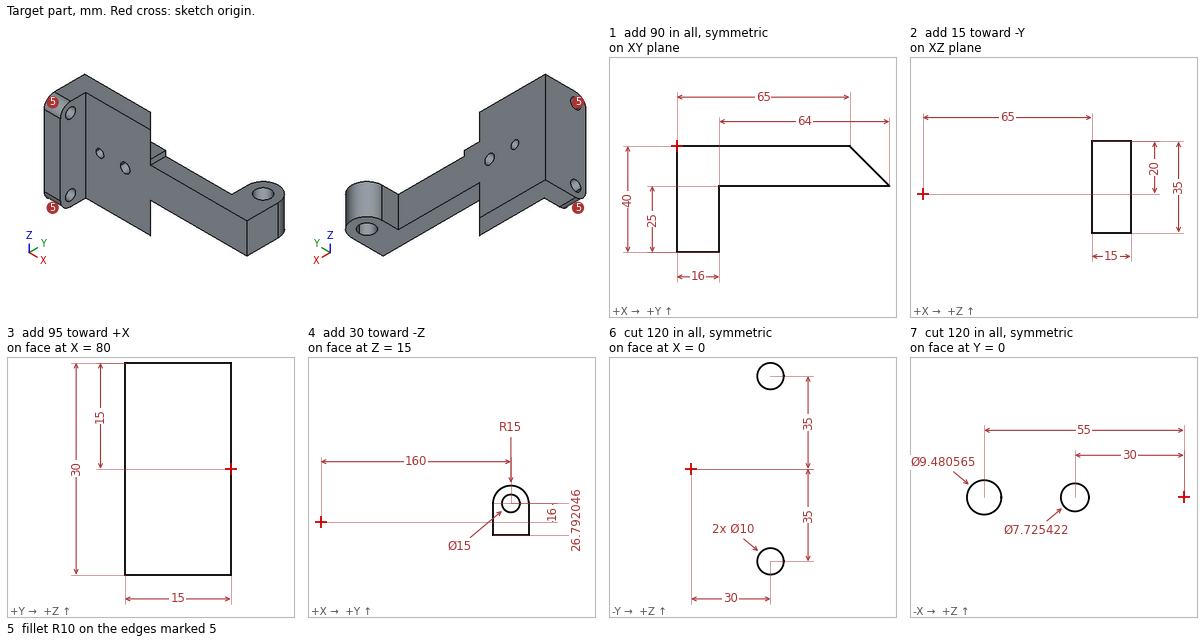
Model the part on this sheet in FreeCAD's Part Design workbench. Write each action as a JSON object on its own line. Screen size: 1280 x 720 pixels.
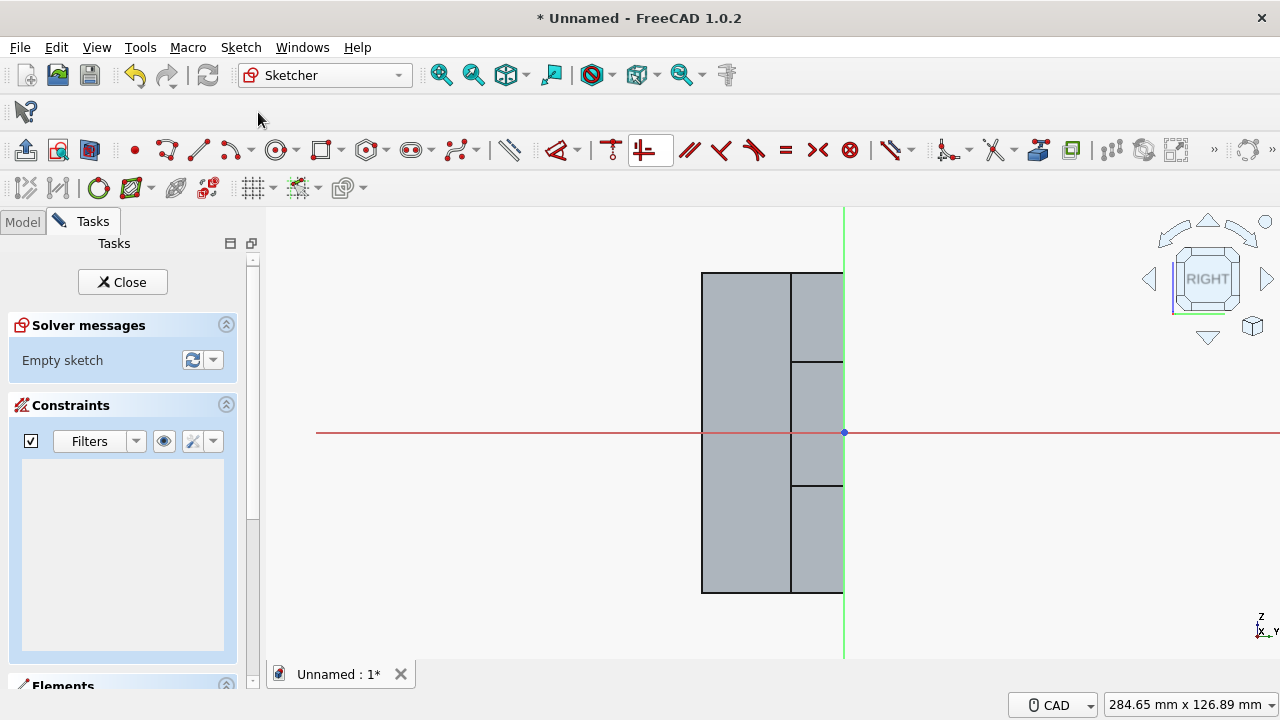
{"action": "scroll", "coordinate": [883, 433], "scroll_direction": "up", "scroll_amount": 5}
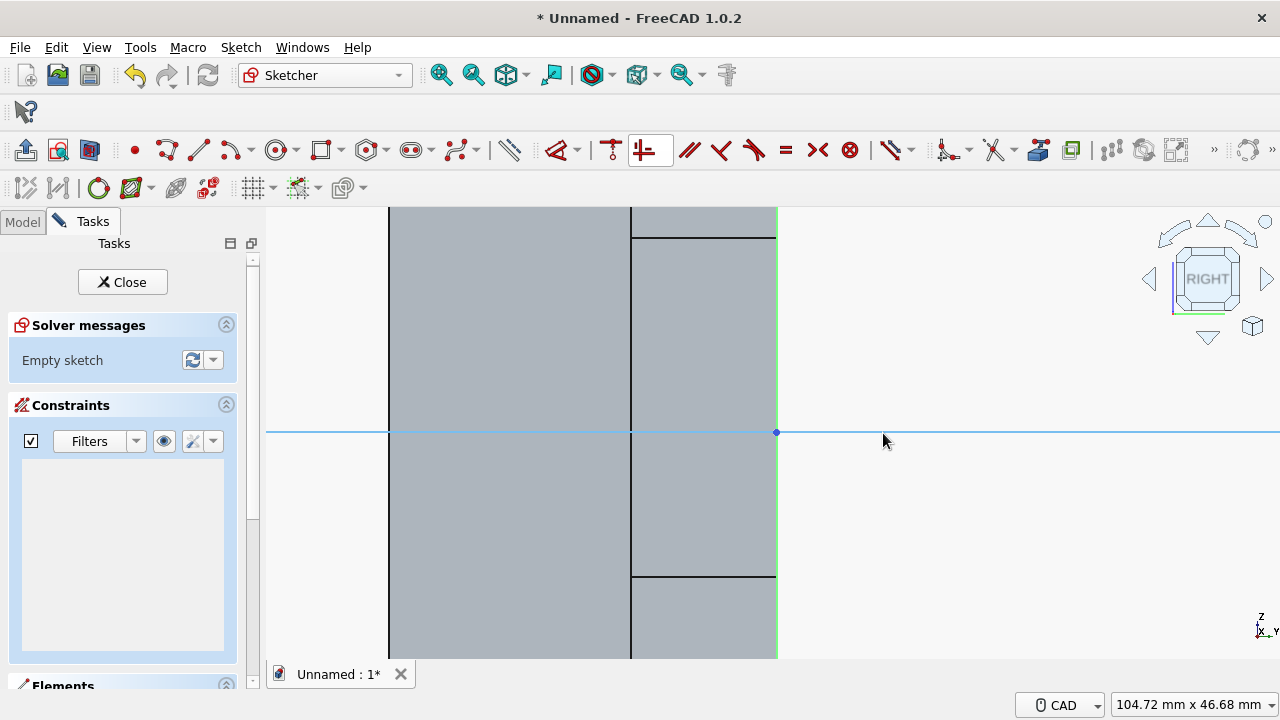
{"action": "left_click", "coordinate": [322, 150]}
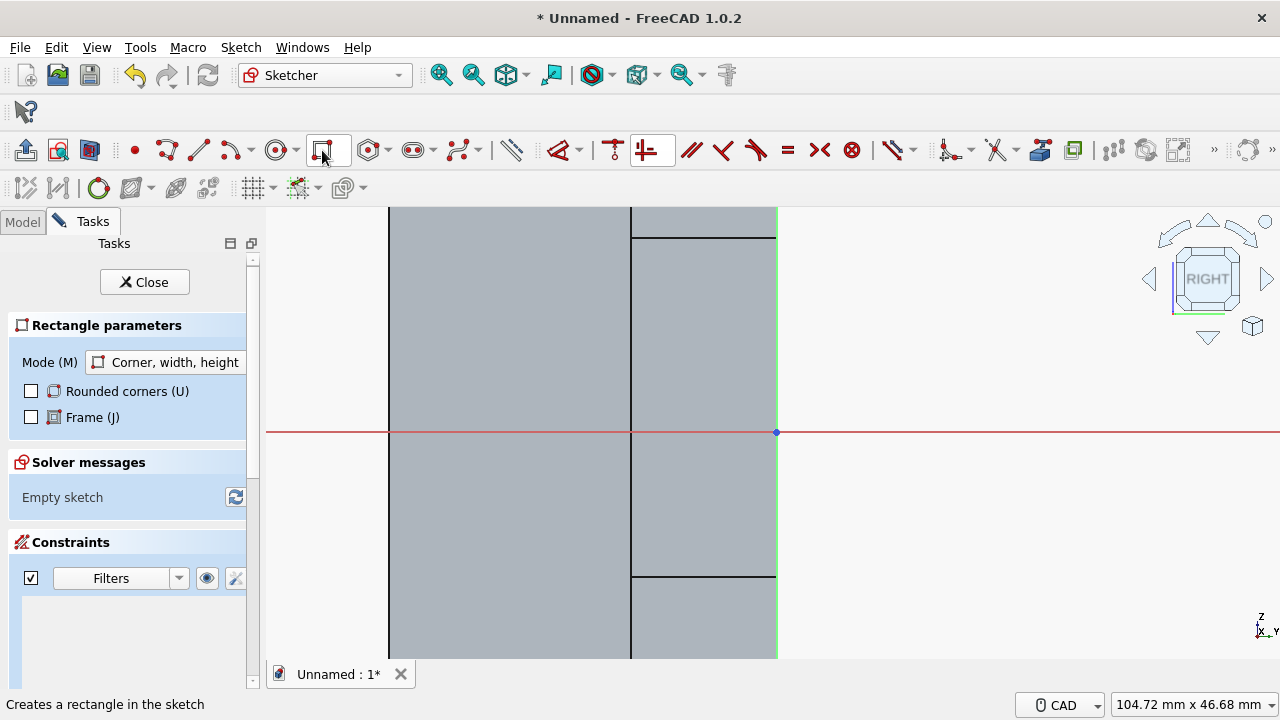
{"action": "left_click", "coordinate": [631, 287]}
{"action": "left_click", "coordinate": [777, 577]}
{"action": "key", "text": "Escape"}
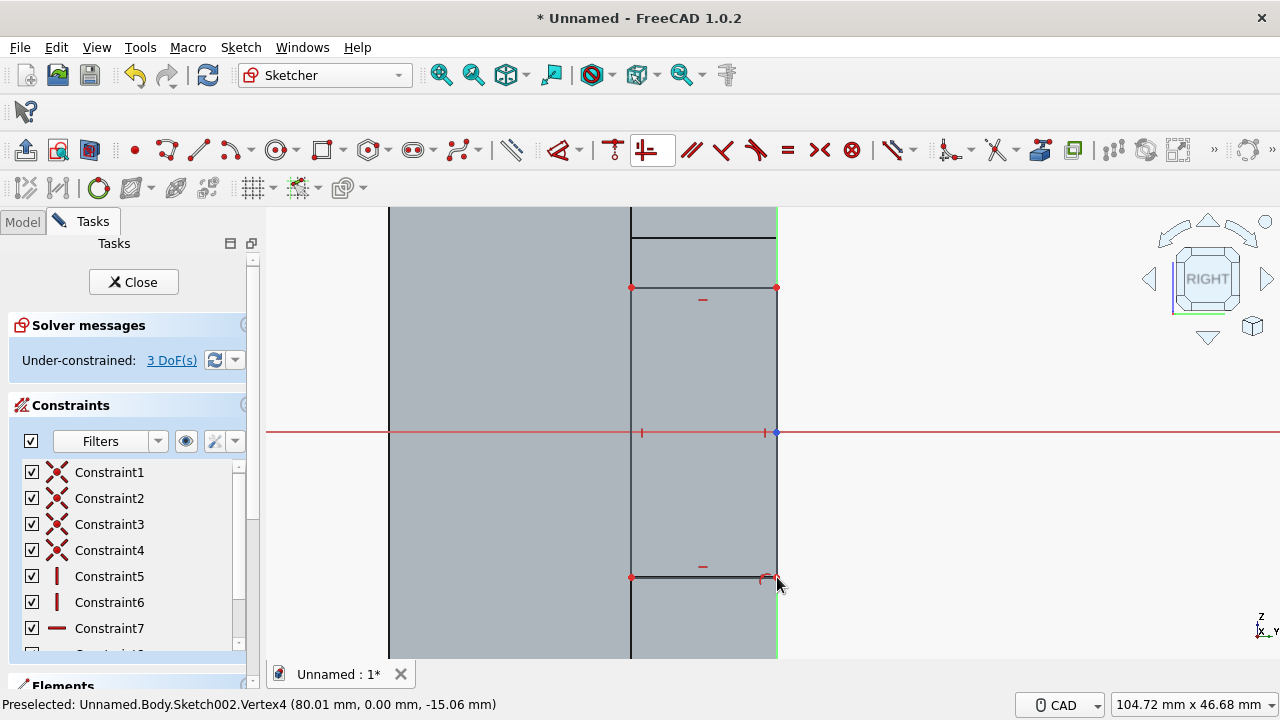
{"action": "left_click", "coordinate": [558, 150]}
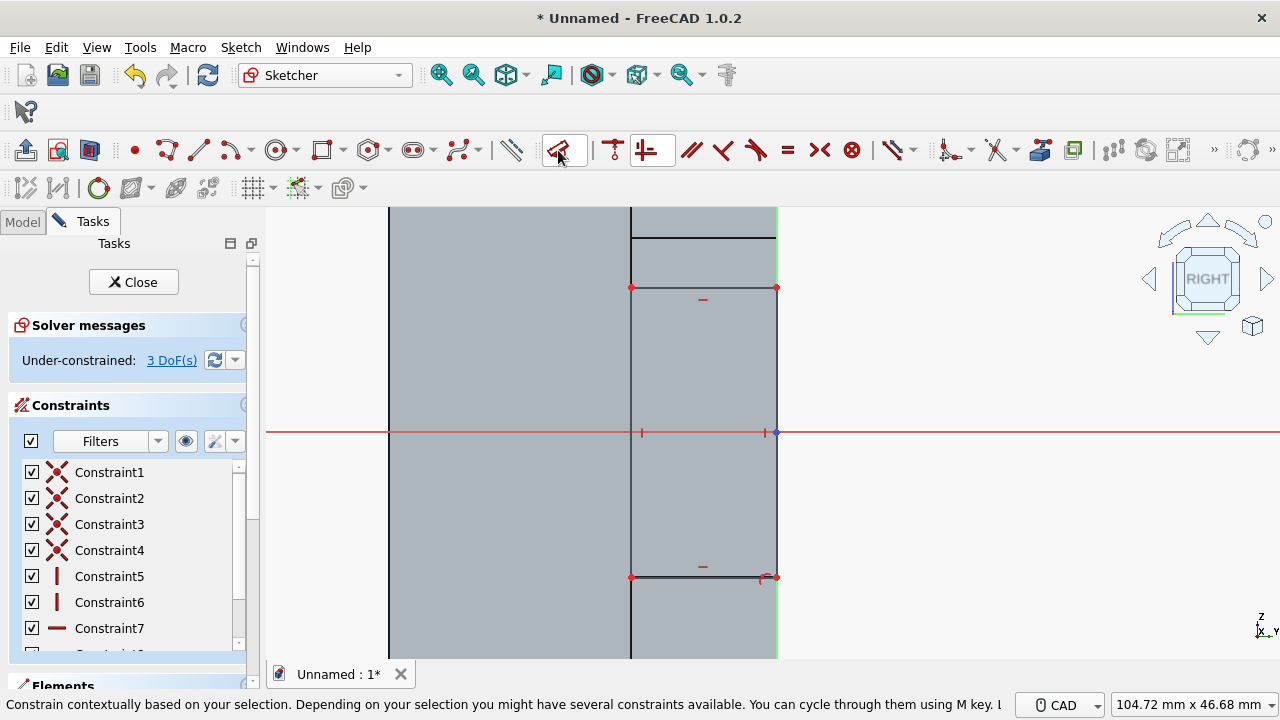
{"action": "left_click", "coordinate": [631, 375]}
{"action": "left_click", "coordinate": [597, 366]}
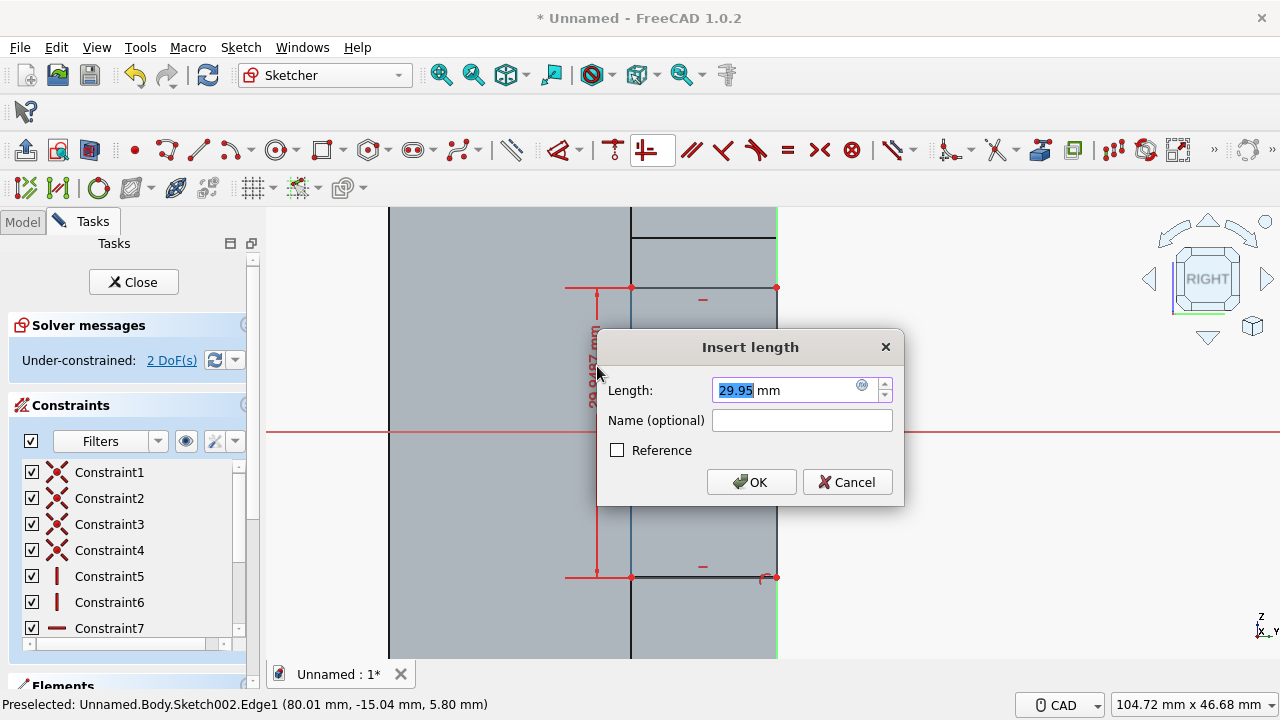
{"action": "type", "text": "30"}
{"action": "key", "text": "Return"}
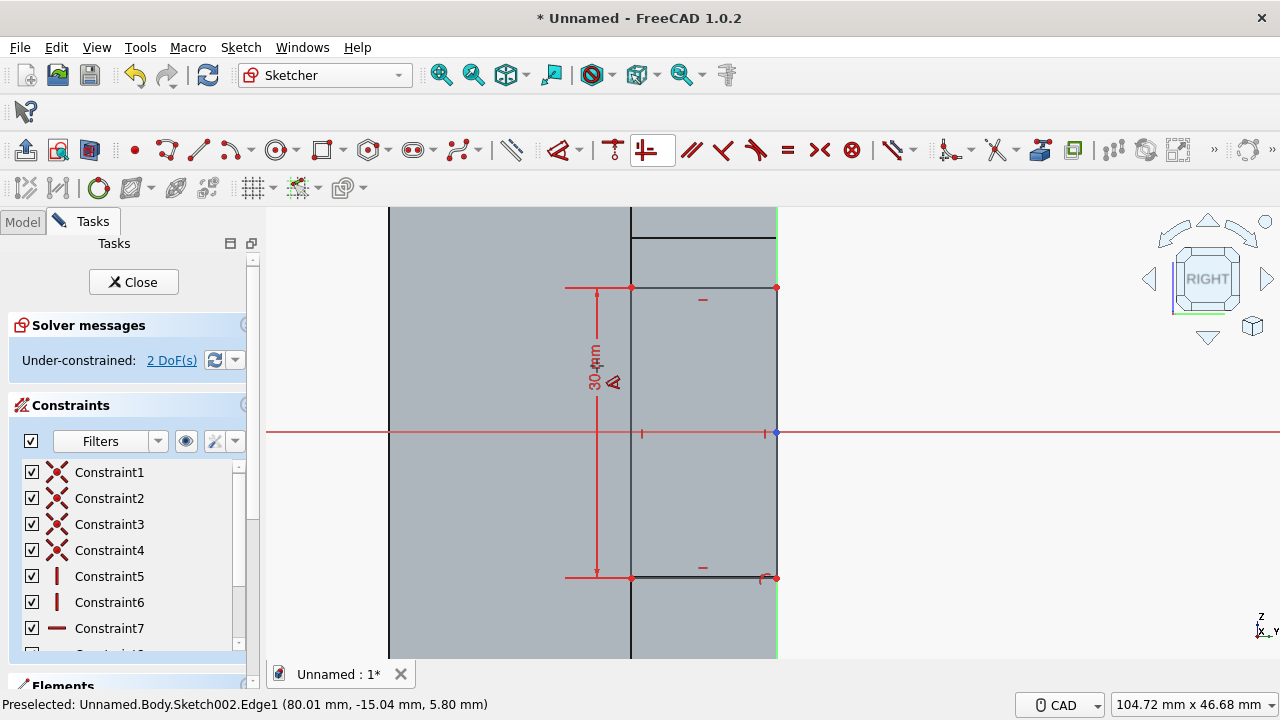
{"action": "left_click", "coordinate": [675, 578]}
{"action": "left_click", "coordinate": [704, 612]}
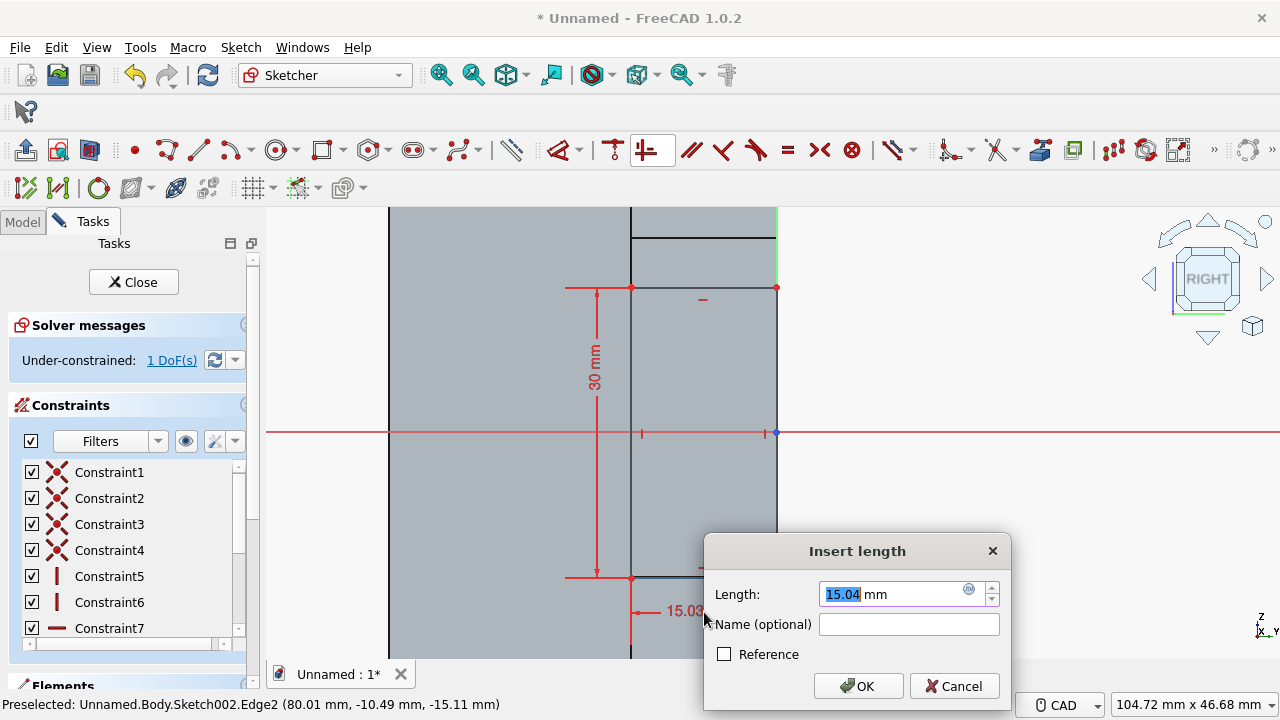
{"action": "type", "text": "15"}
{"action": "key", "text": "Return"}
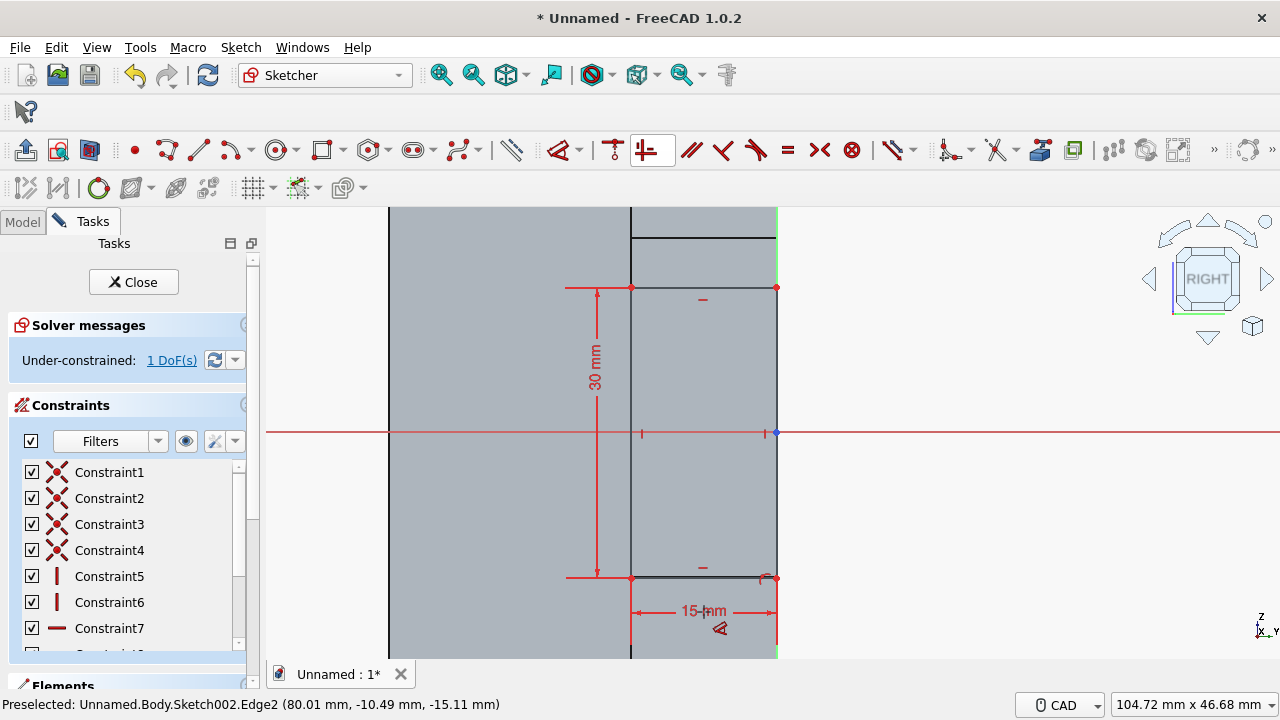
{"action": "left_click", "coordinate": [631, 288]}
{"action": "left_click", "coordinate": [811, 360]}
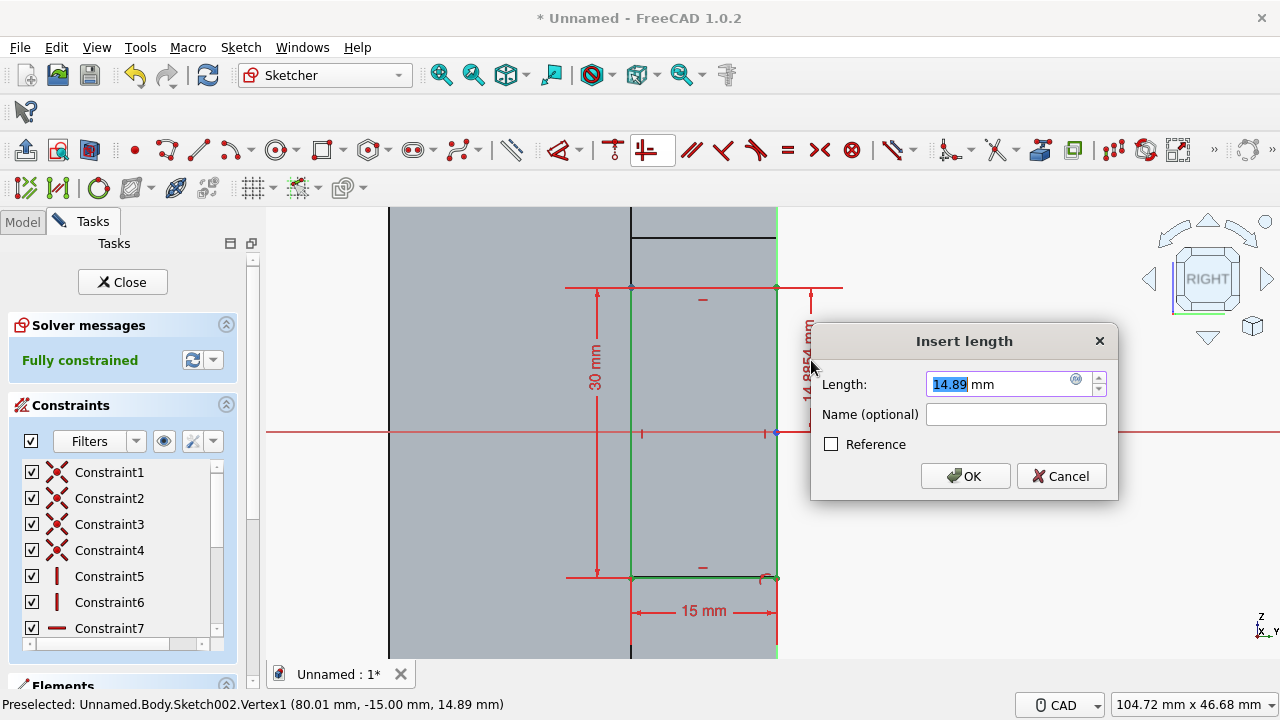
{"action": "type", "text": "15"}
{"action": "key", "text": "Return"}
{"action": "key", "text": "Escape"}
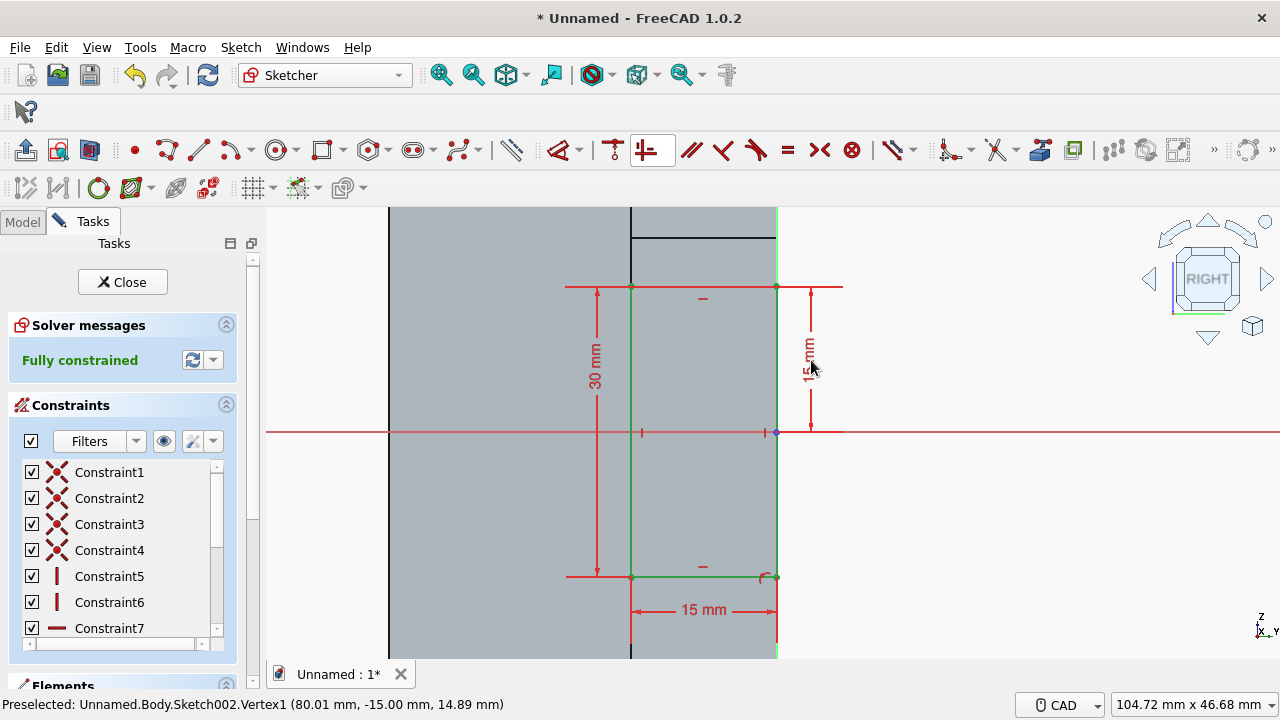
{"action": "left_click", "coordinate": [123, 282]}